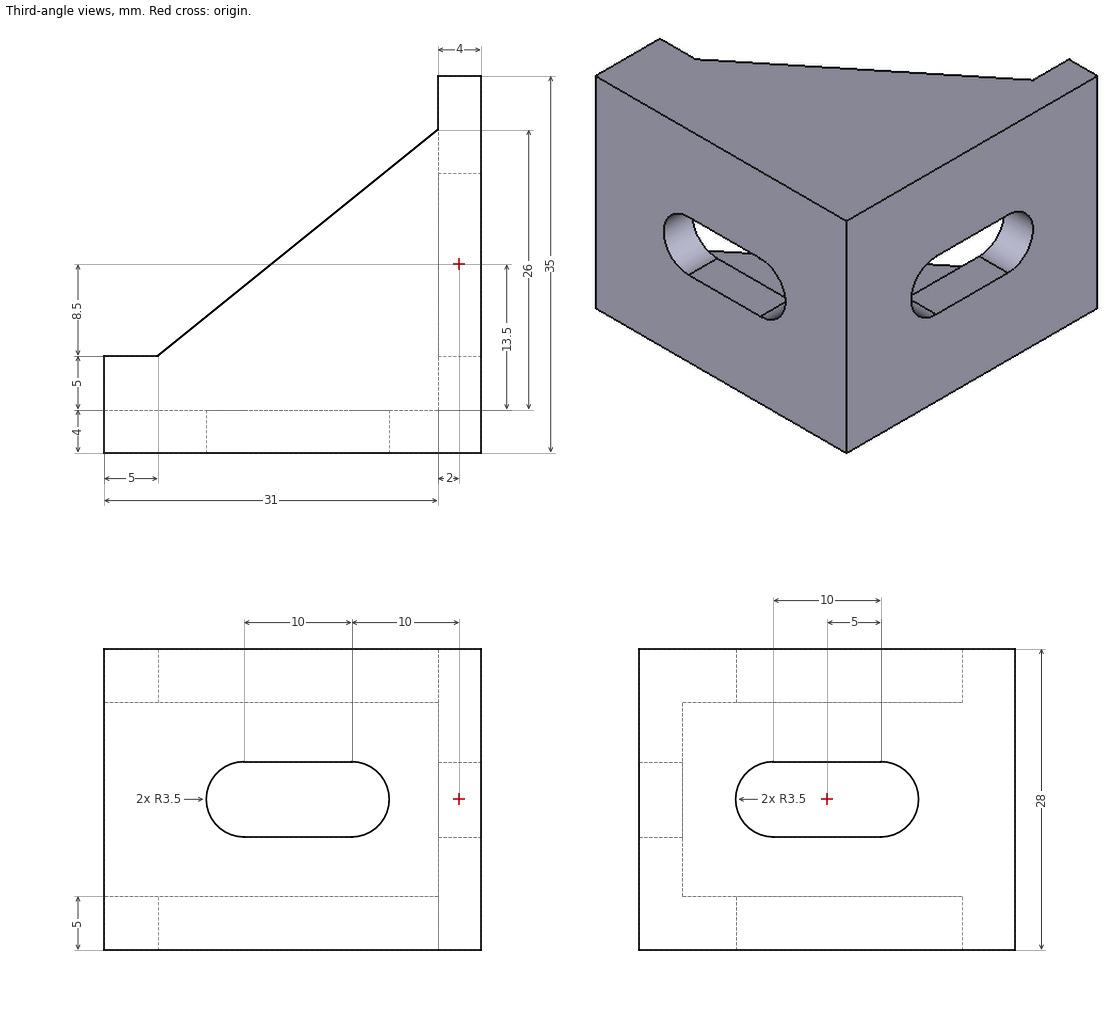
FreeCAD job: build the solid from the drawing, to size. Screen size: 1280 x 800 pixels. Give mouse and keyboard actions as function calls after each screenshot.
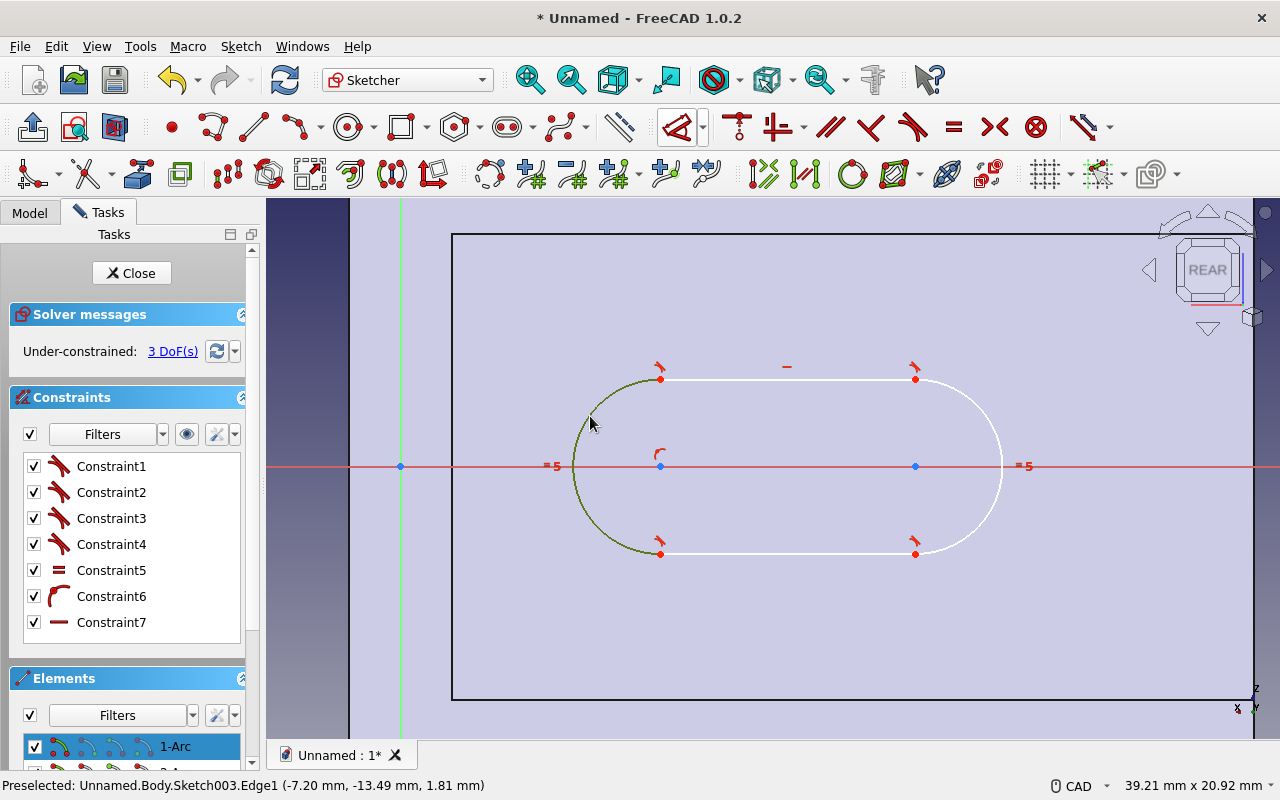
key(k)
key(r)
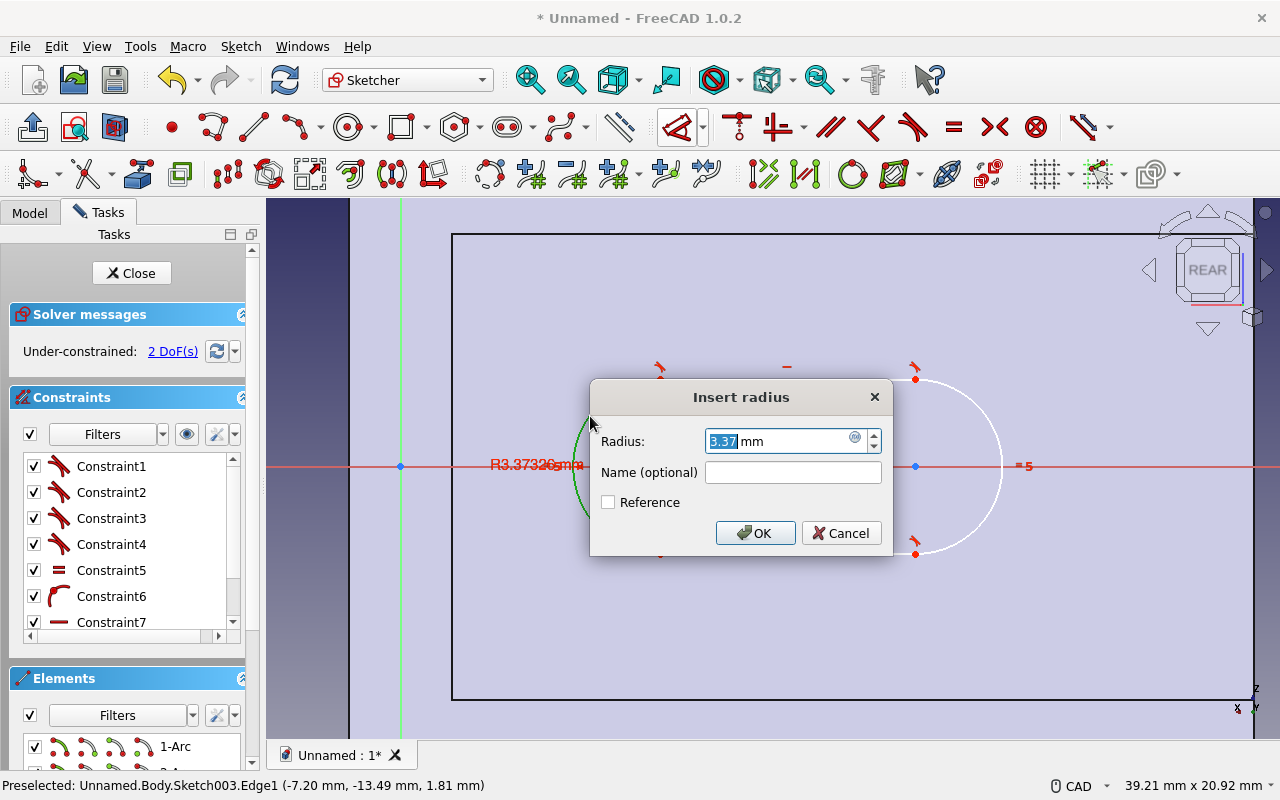
text(3.5)
key(Return)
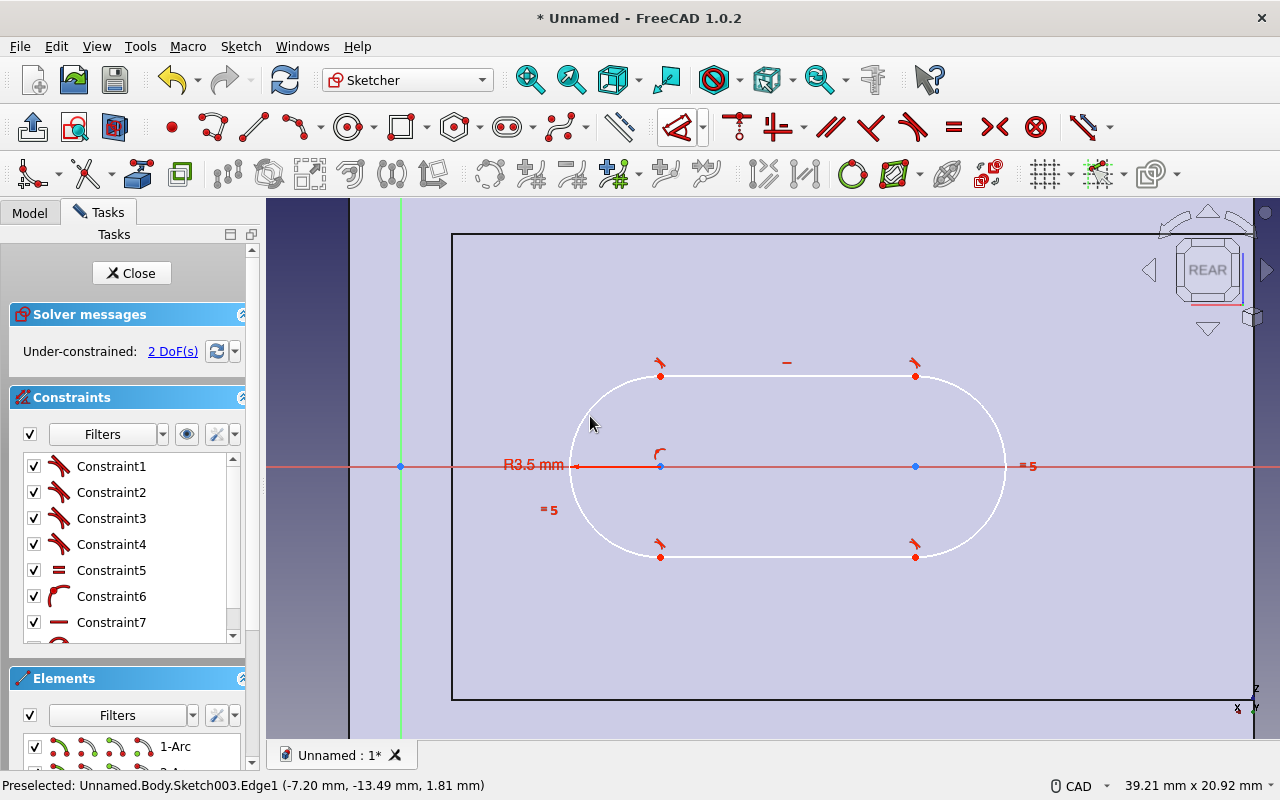
click(737, 376)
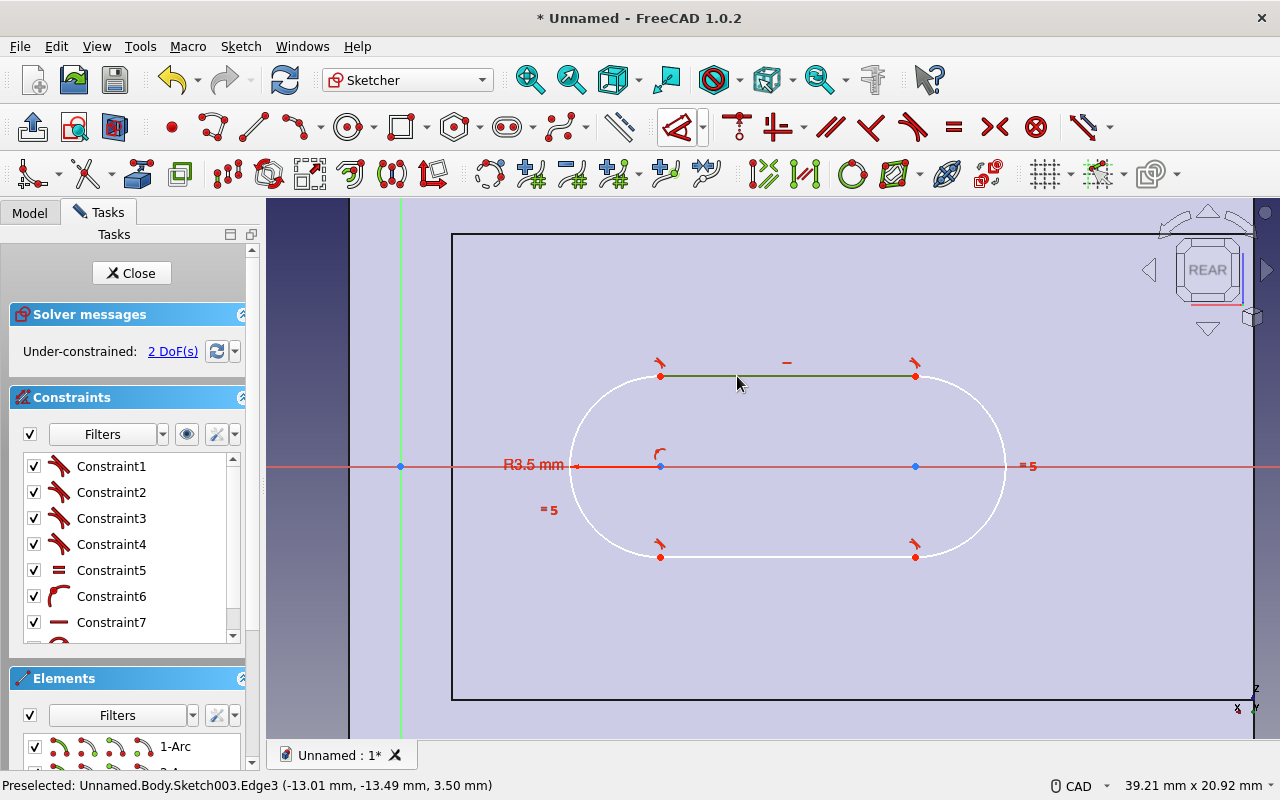
key(l)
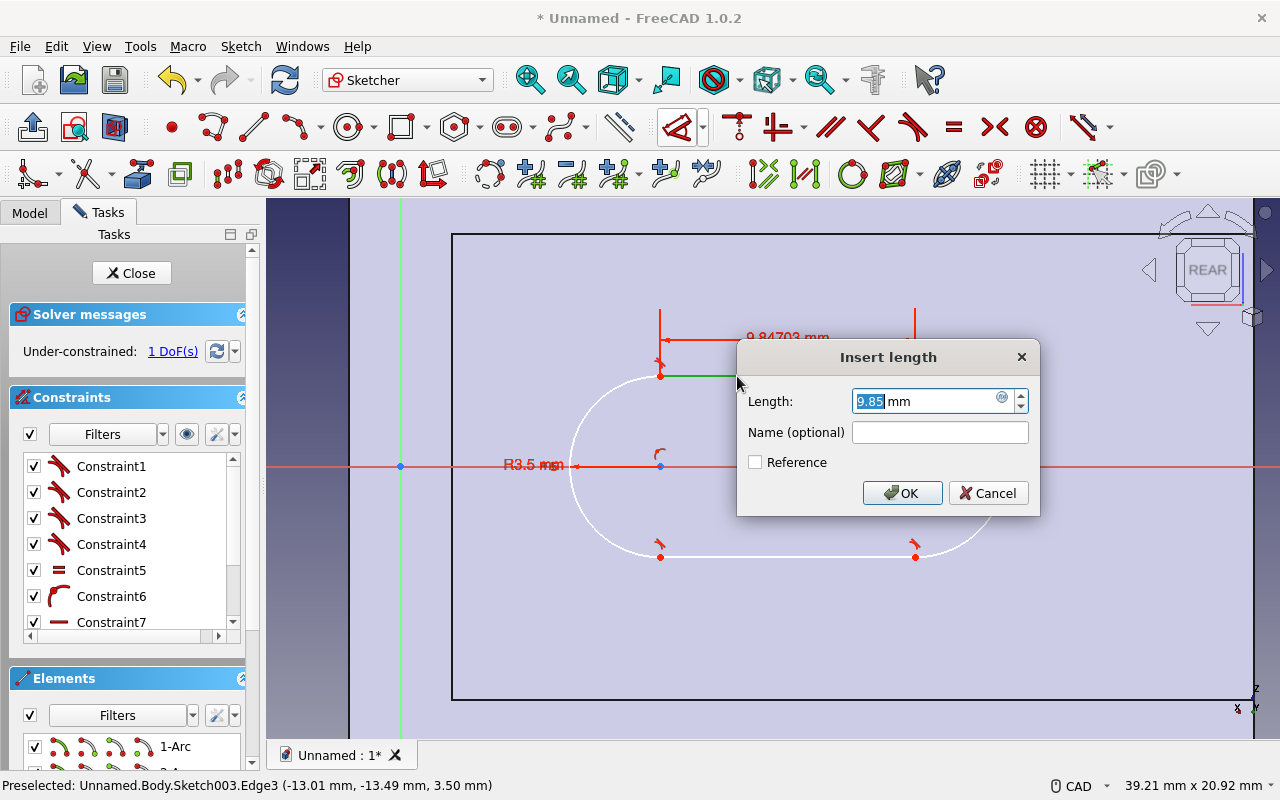
text(10)
key(Return)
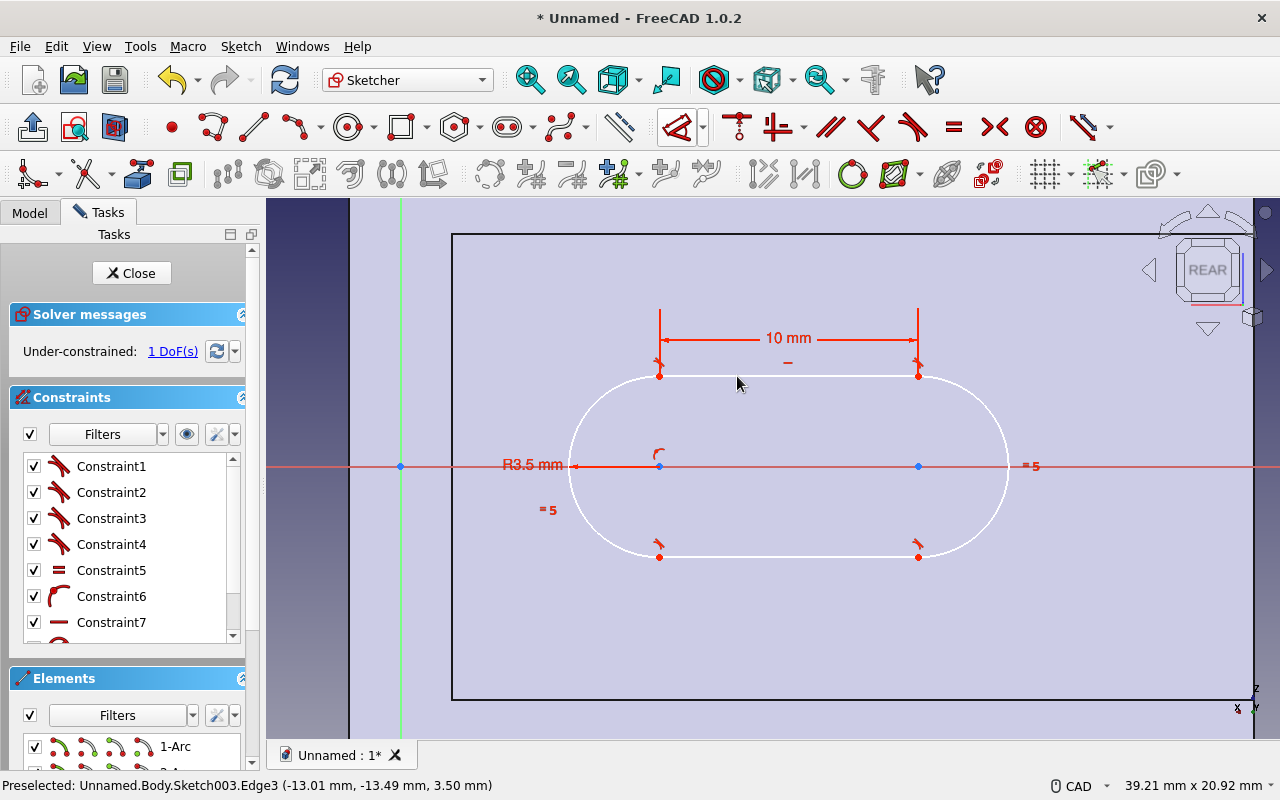
click(660, 376)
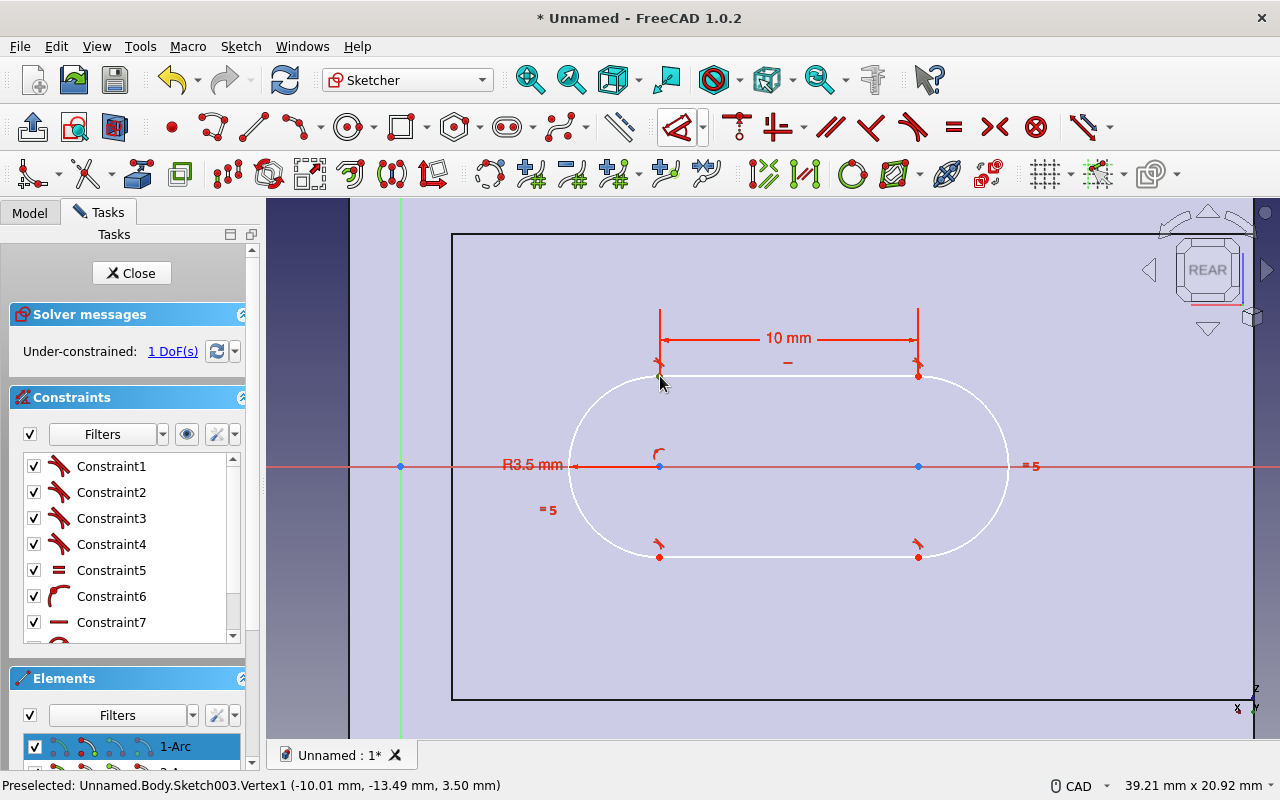
key(l)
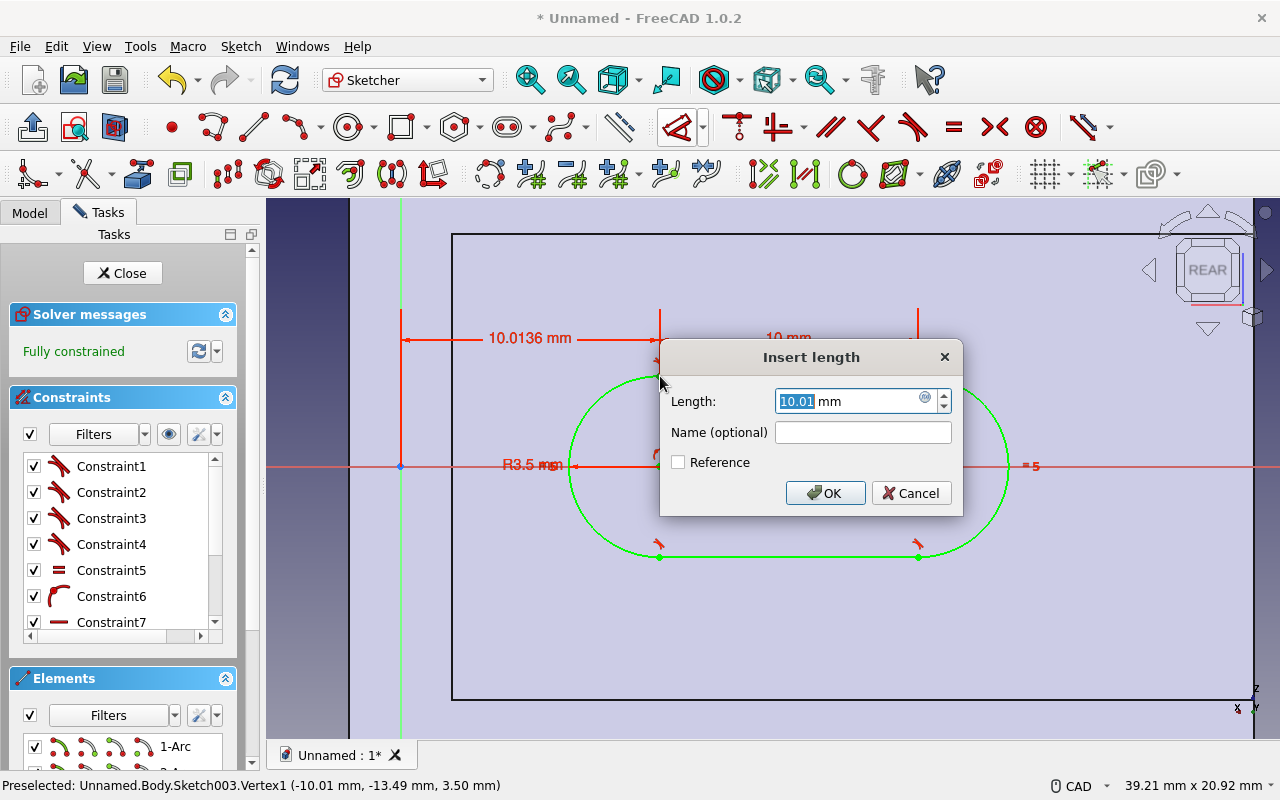
text(10)
key(Return)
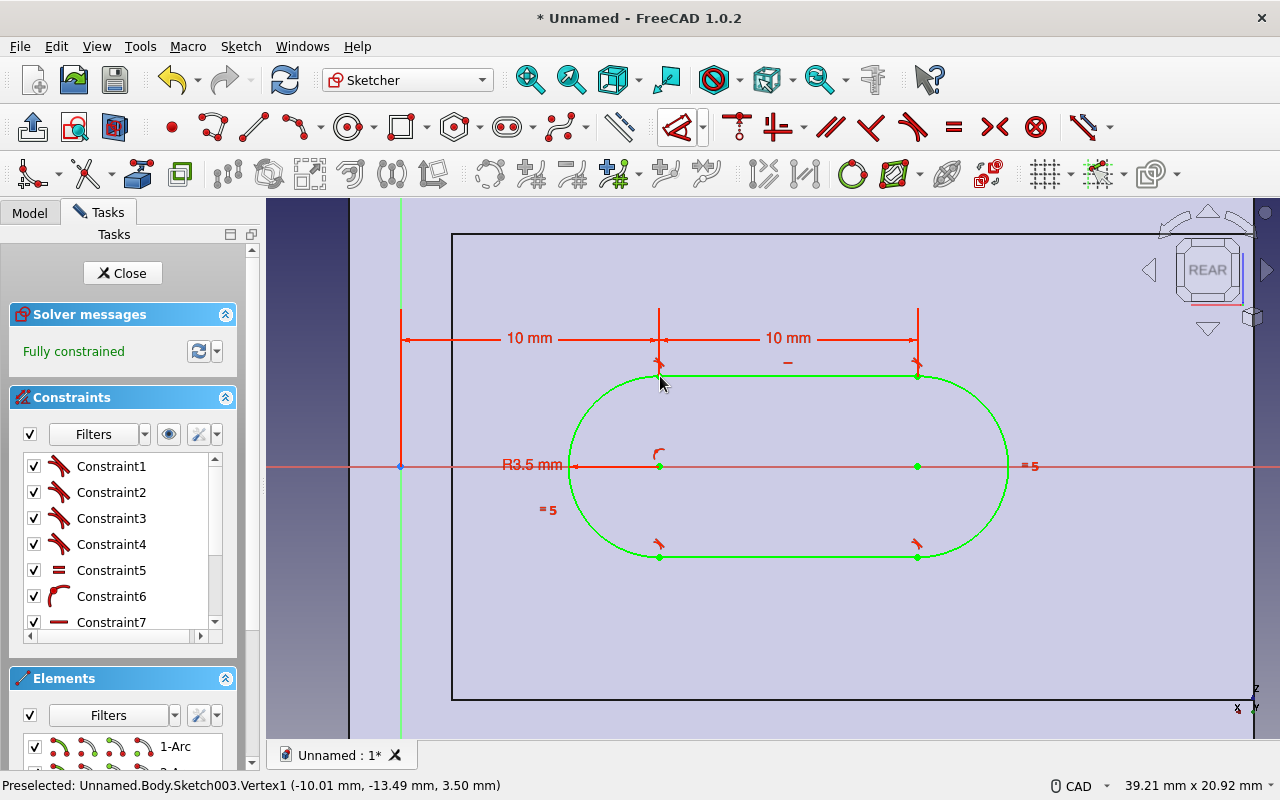
click(123, 273)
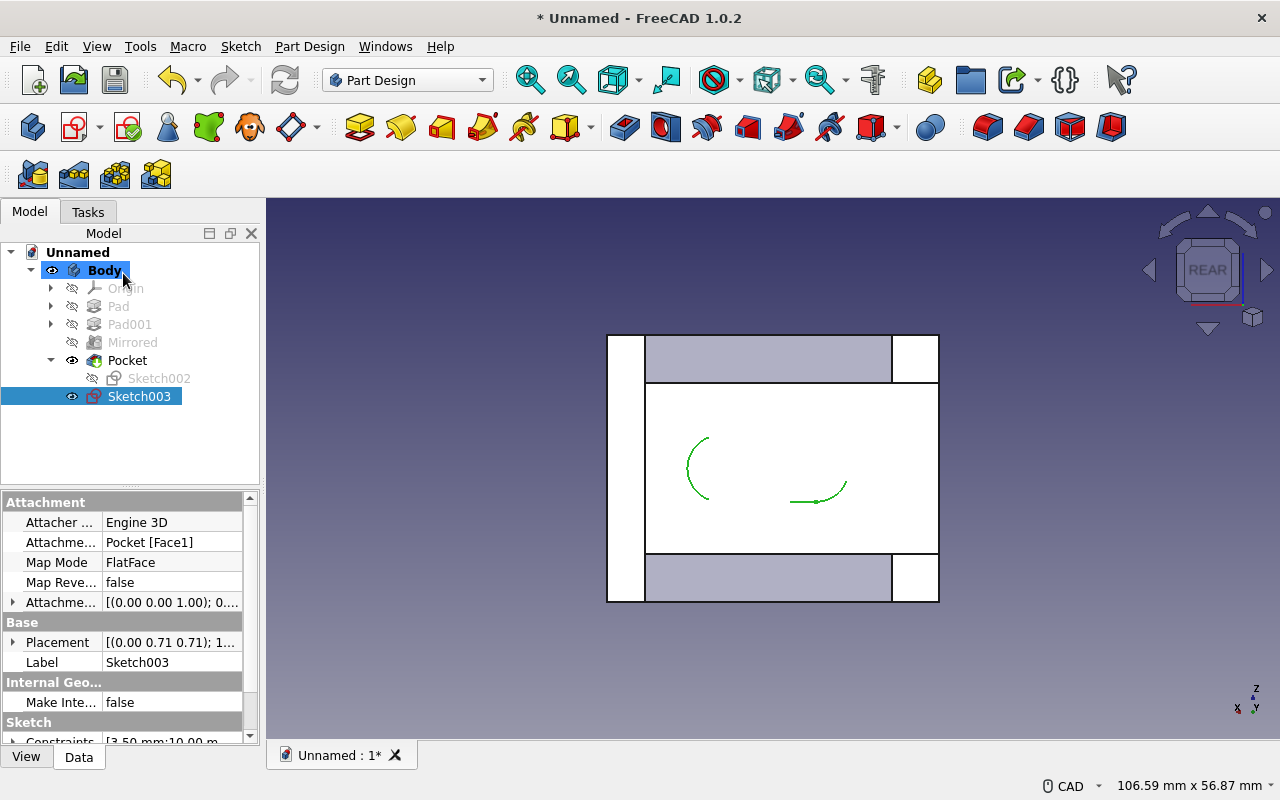
click(625, 128)